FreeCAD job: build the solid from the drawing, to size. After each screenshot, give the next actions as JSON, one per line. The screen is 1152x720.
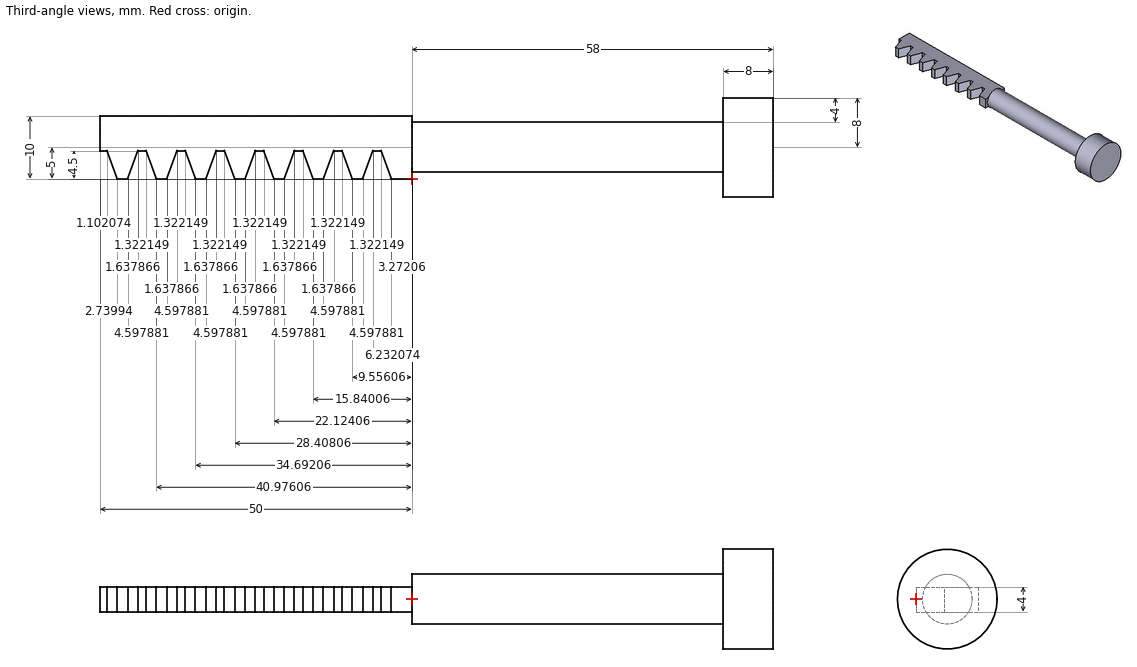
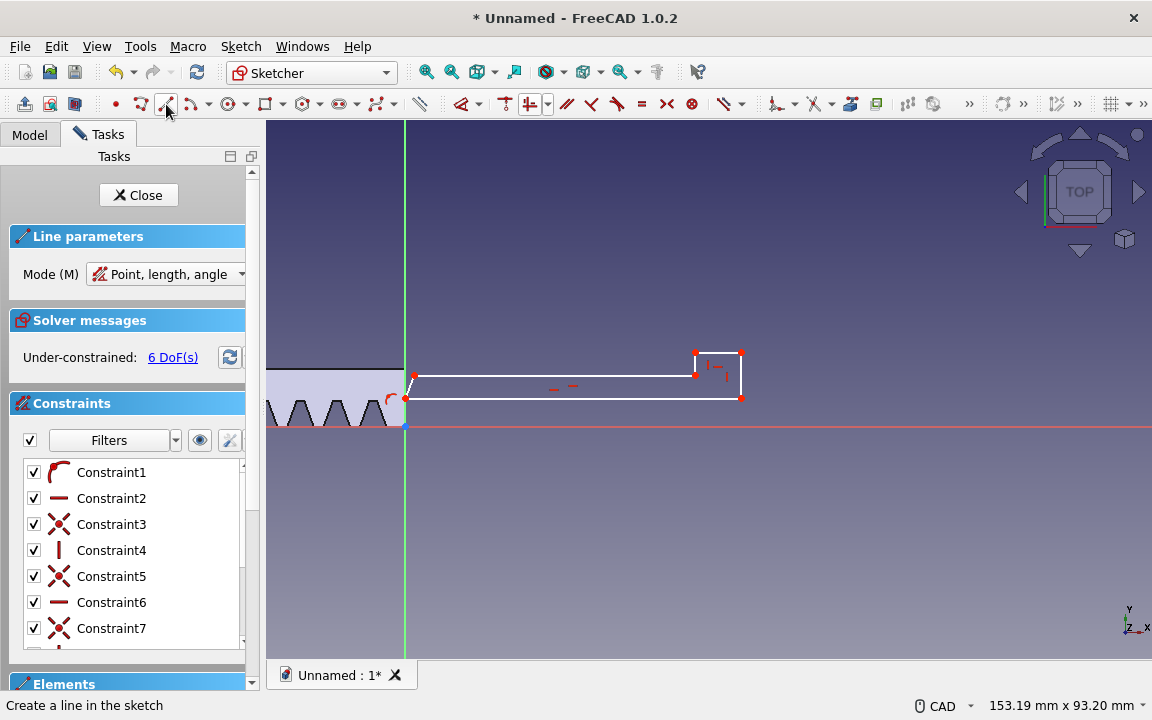
{"action": "left_click", "coordinate": [774, 398]}
{"action": "left_click", "coordinate": [875, 398]}
{"action": "key", "text": "Escape"}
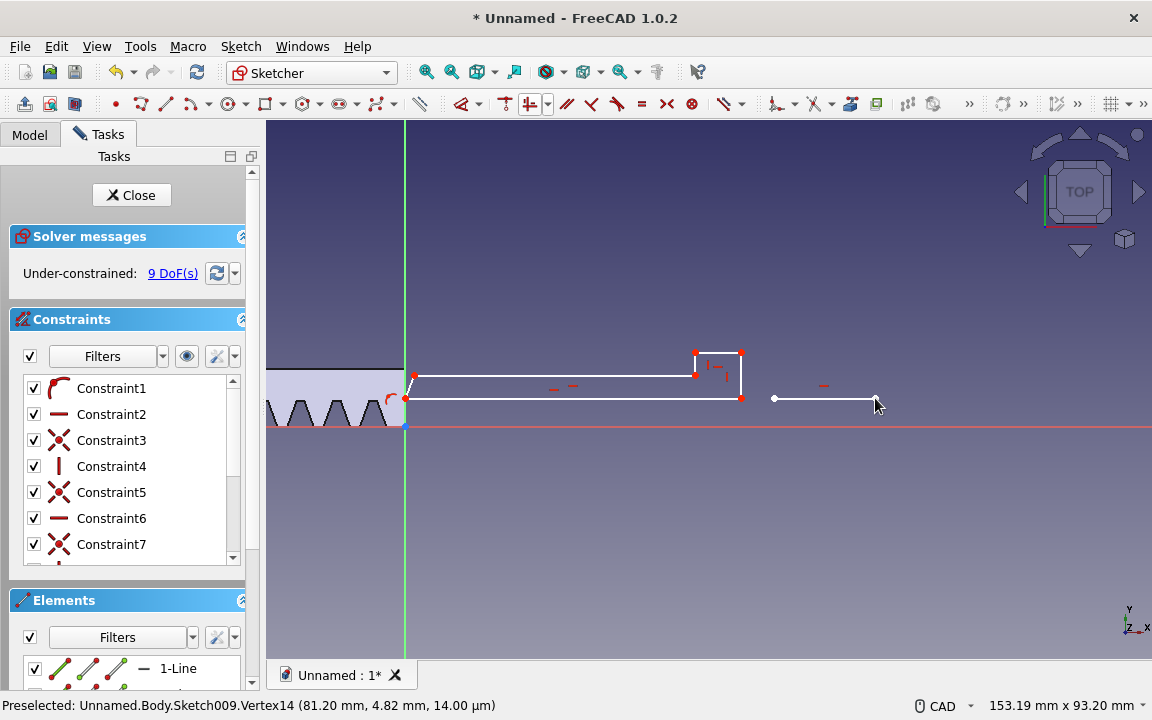
{"action": "left_click", "coordinate": [804, 399]}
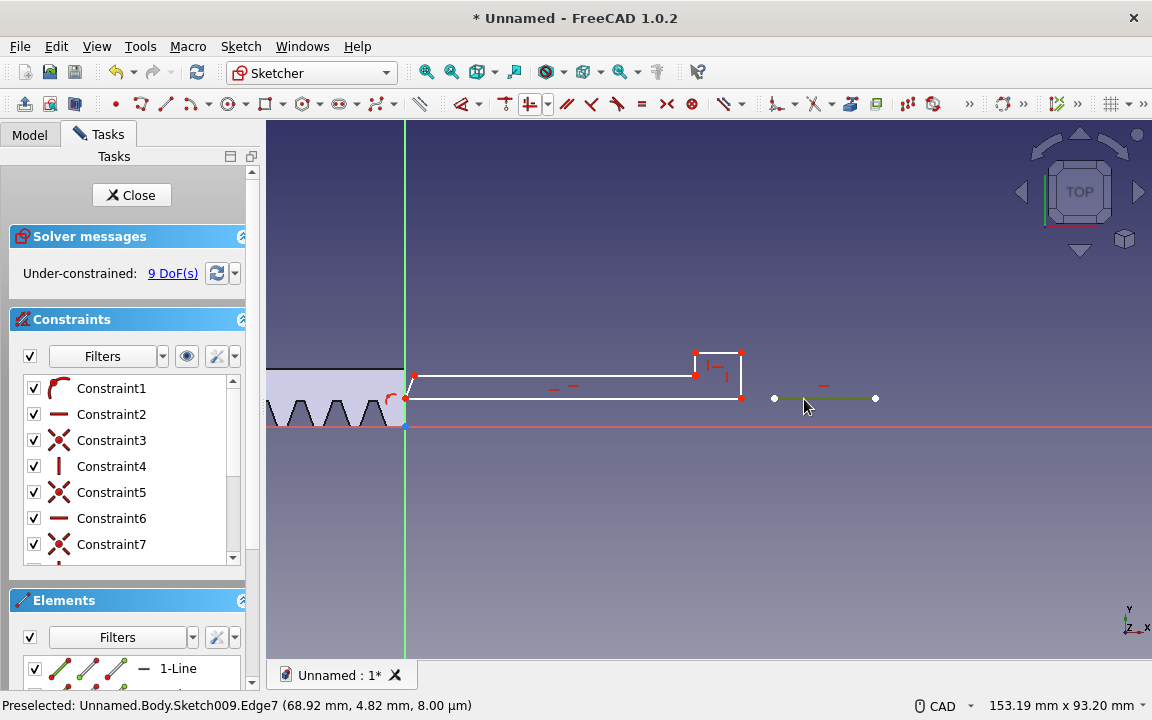
{"action": "left_click", "coordinate": [420, 104]}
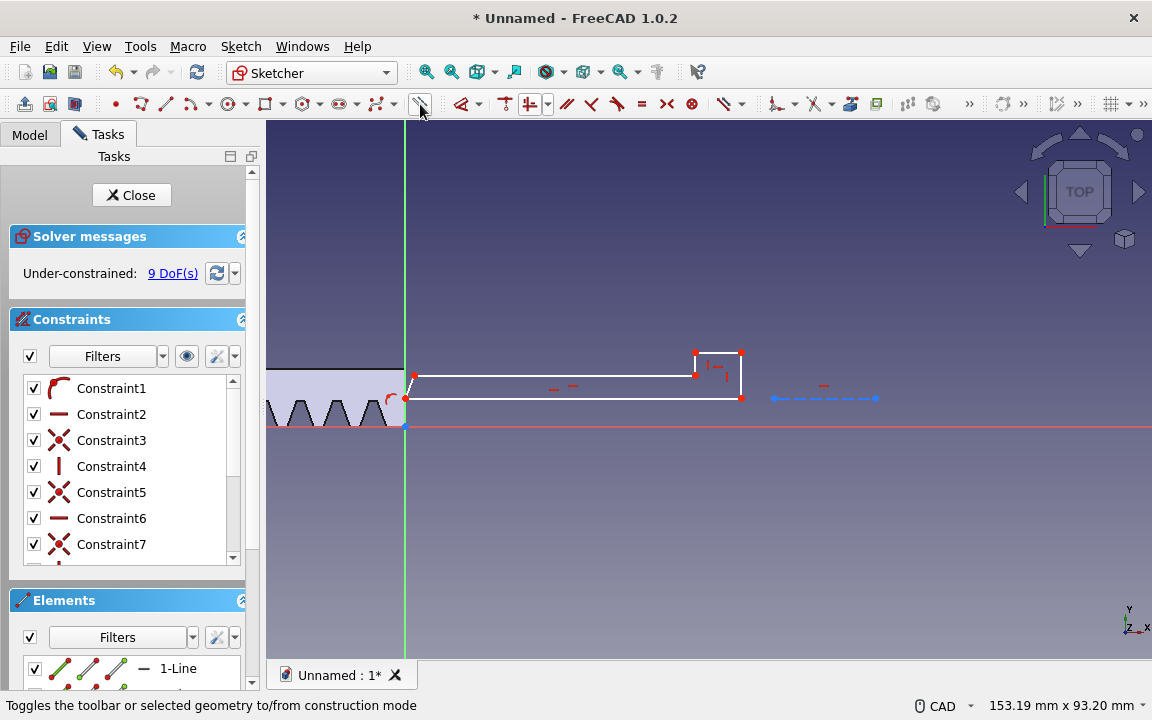
{"action": "scroll", "coordinate": [409, 390], "scroll_direction": "up", "scroll_amount": 3}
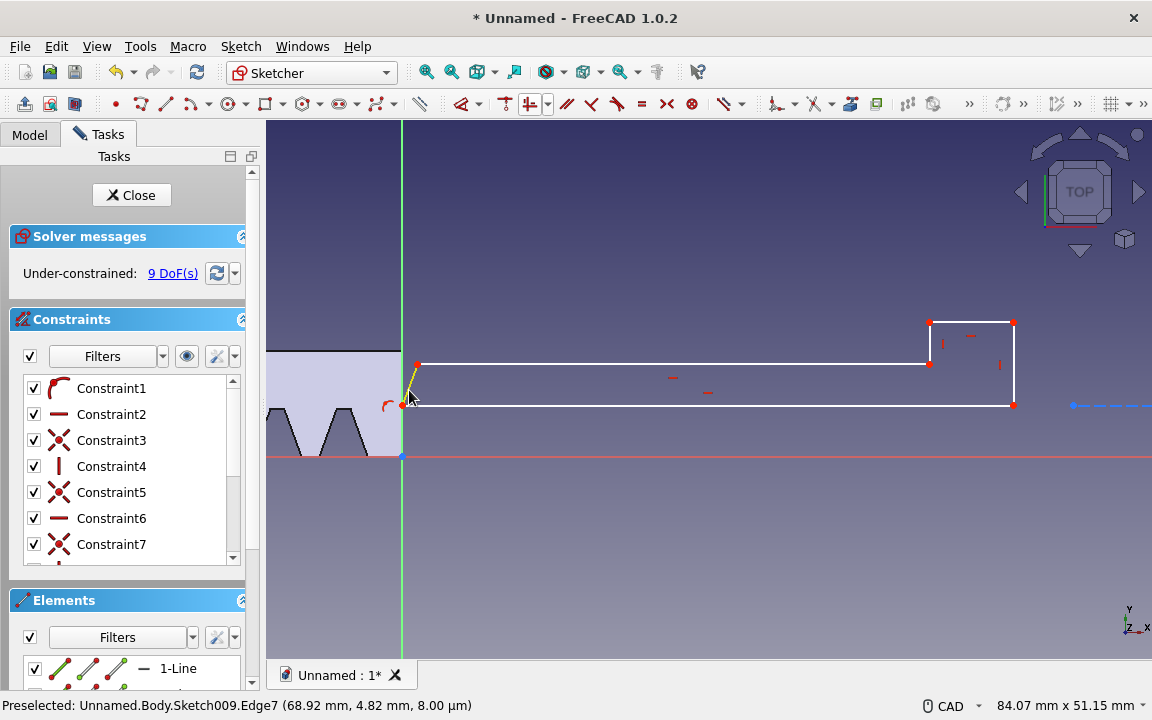
{"action": "left_click", "coordinate": [409, 389]}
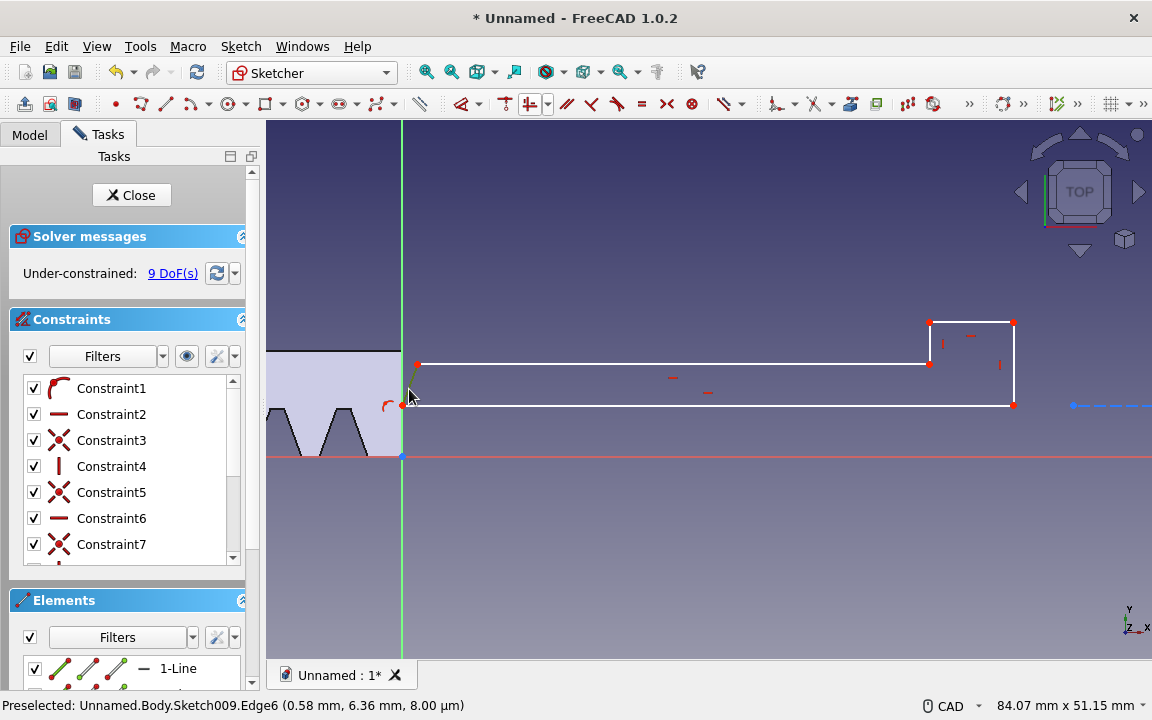
{"action": "left_click", "coordinate": [548, 104]}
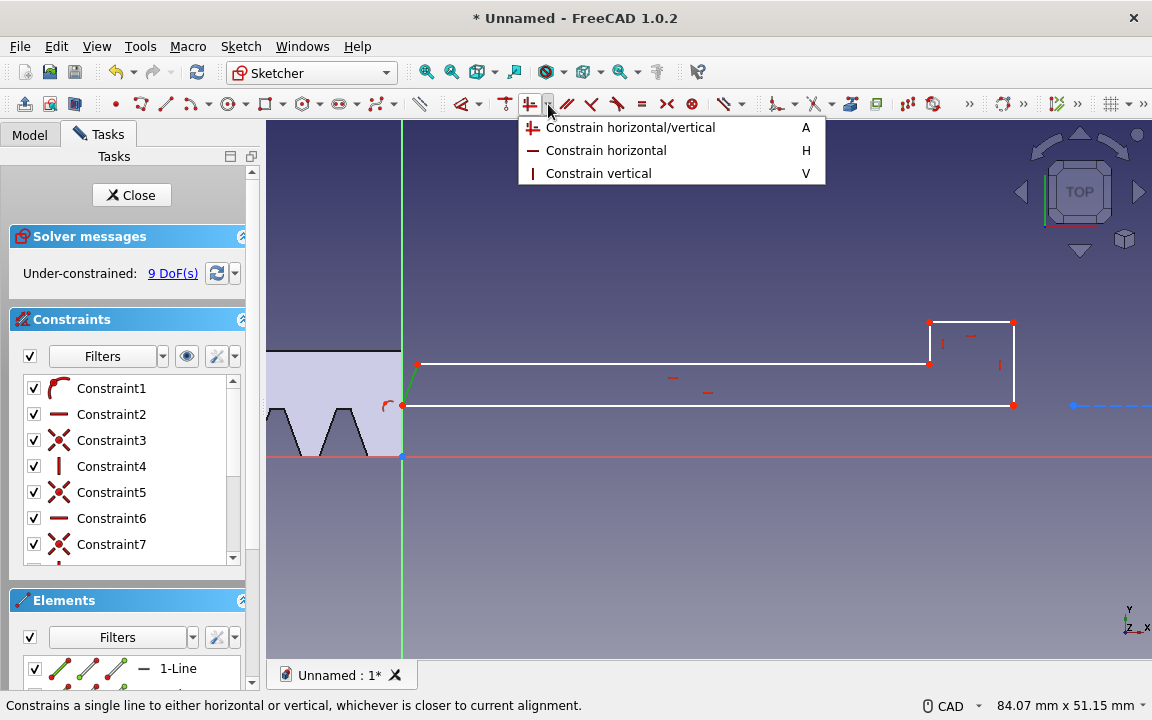
{"action": "left_click", "coordinate": [672, 174]}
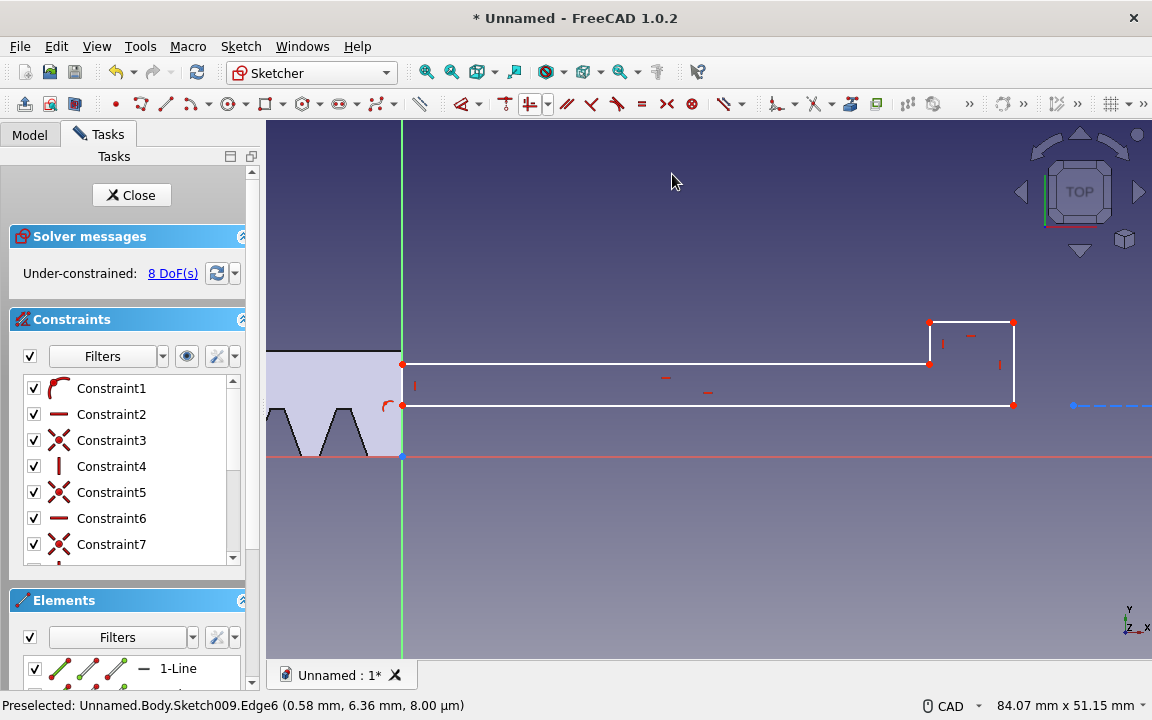
{"action": "left_click", "coordinate": [460, 104]}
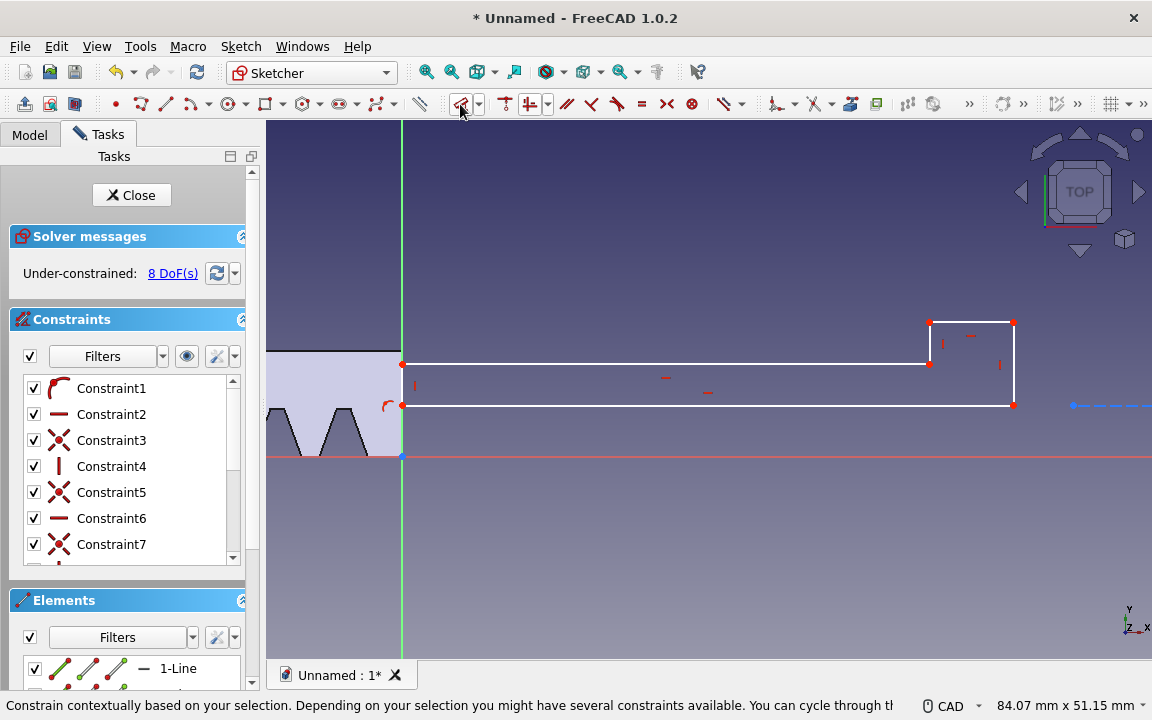
{"action": "scroll", "coordinate": [410, 391], "scroll_direction": "down", "scroll_amount": 3}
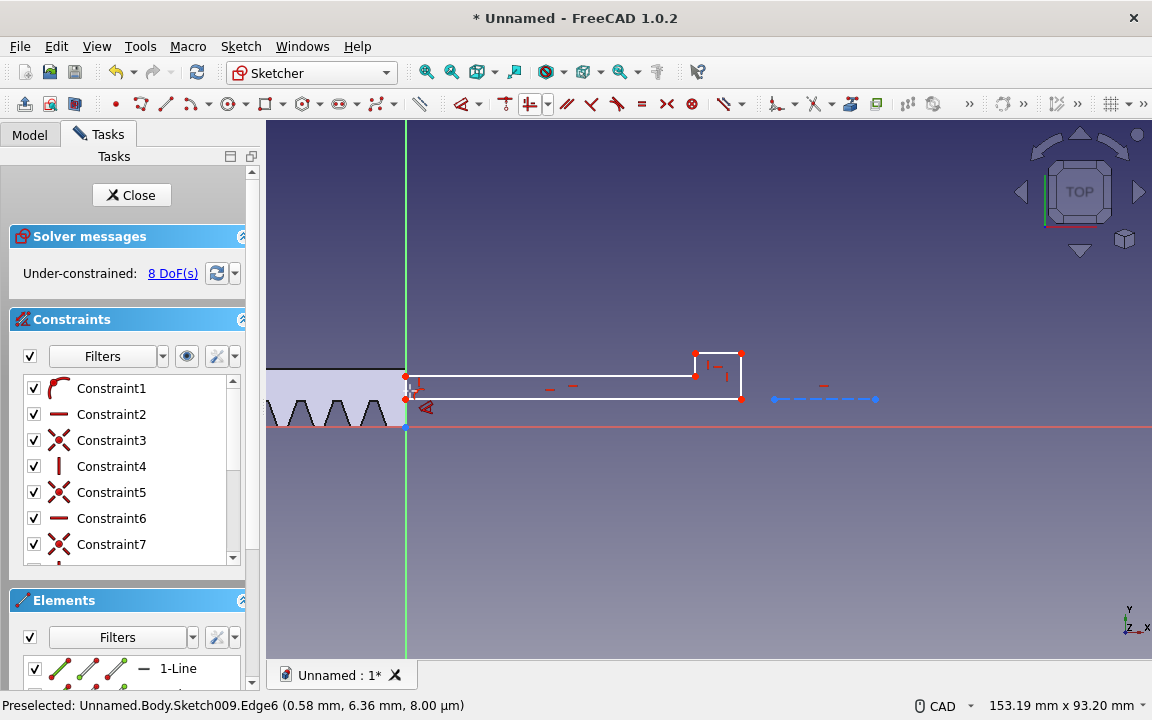
{"action": "left_click", "coordinate": [741, 386]}
{"action": "left_click", "coordinate": [775, 376]}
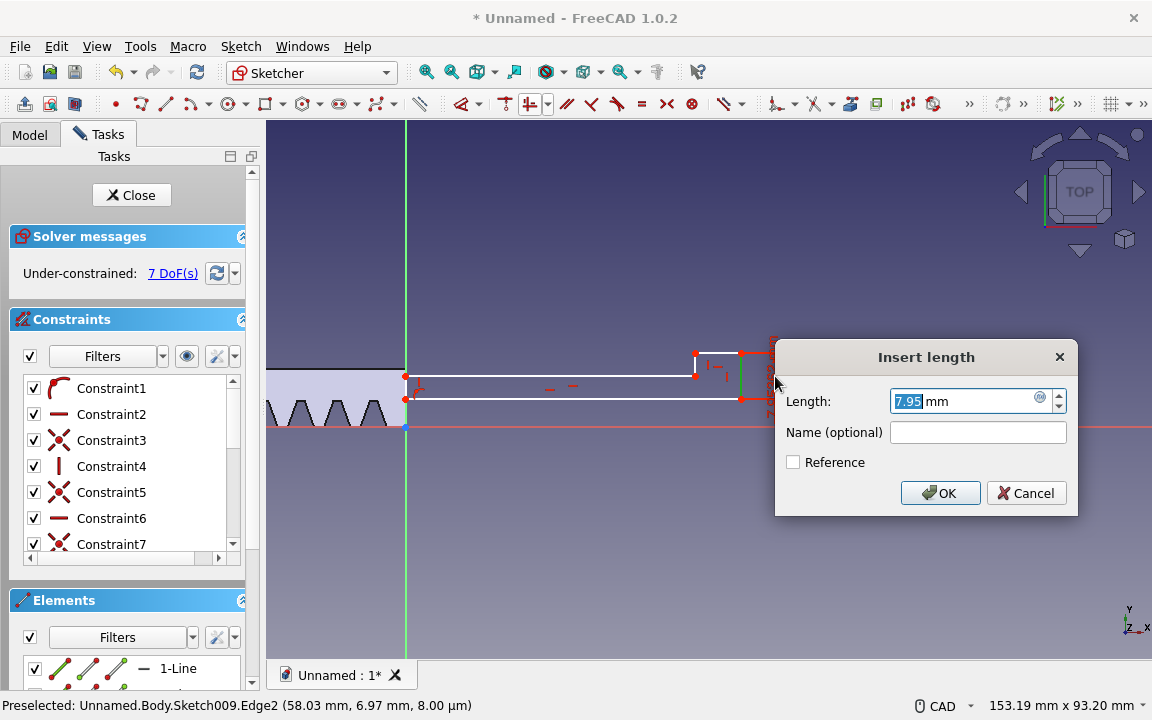
{"action": "type", "text": "8"}
{"action": "key", "text": "Return"}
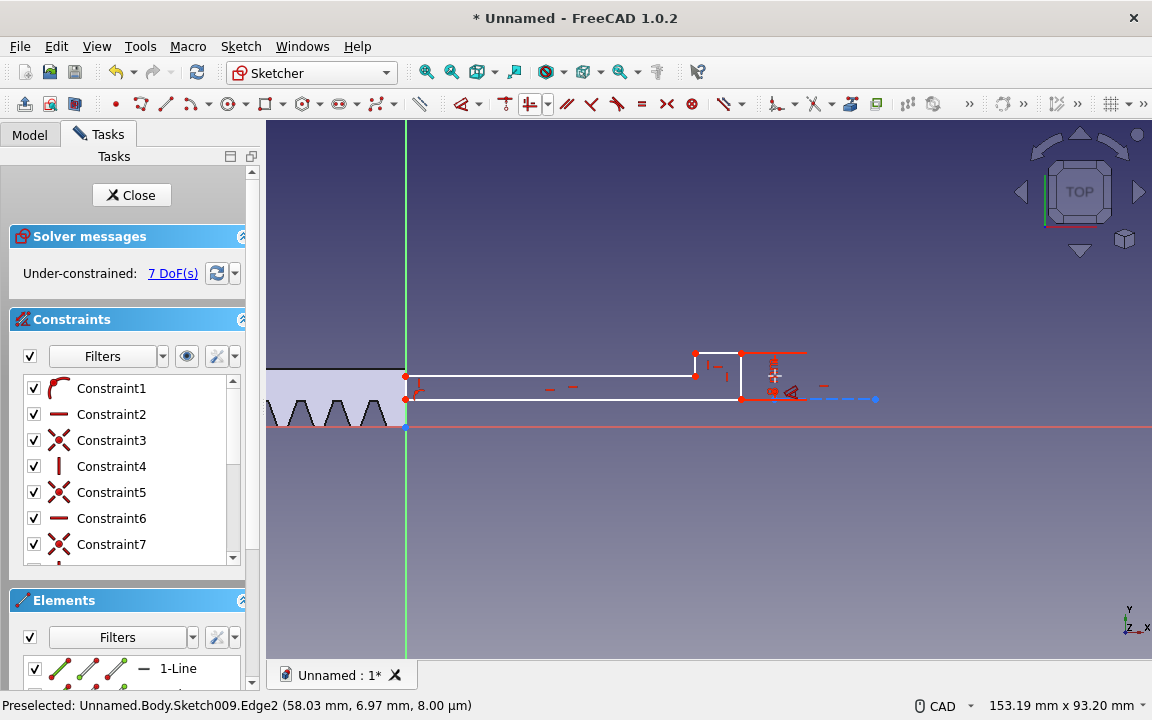
{"action": "left_click", "coordinate": [728, 353]}
{"action": "left_click", "coordinate": [718, 319]}